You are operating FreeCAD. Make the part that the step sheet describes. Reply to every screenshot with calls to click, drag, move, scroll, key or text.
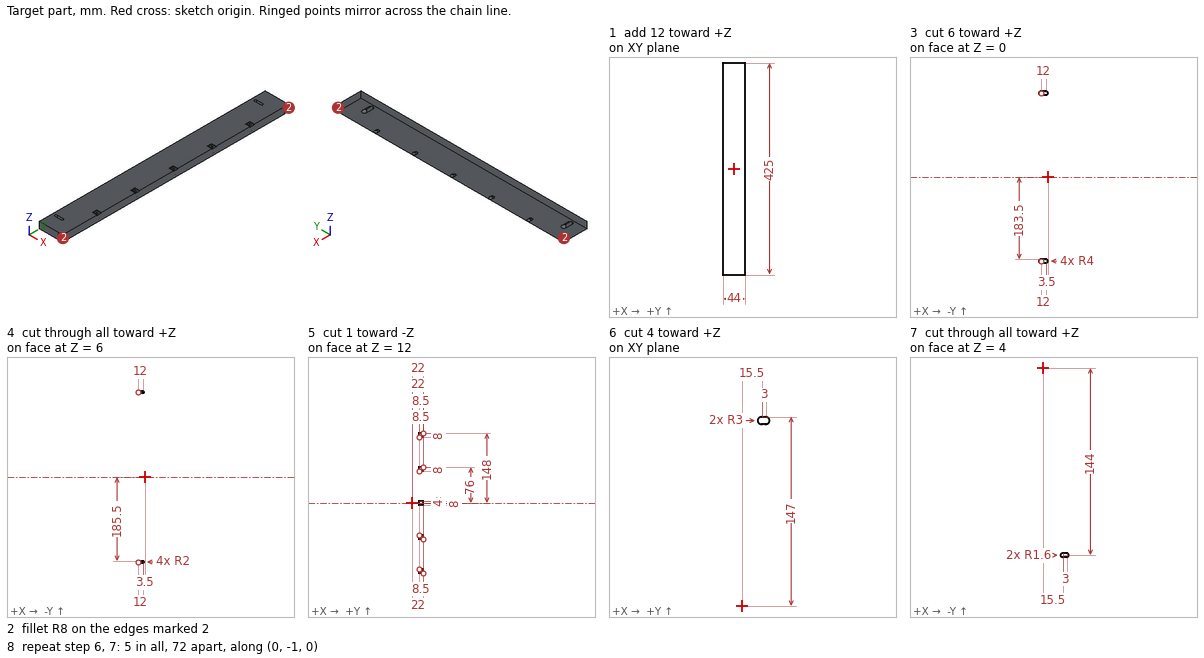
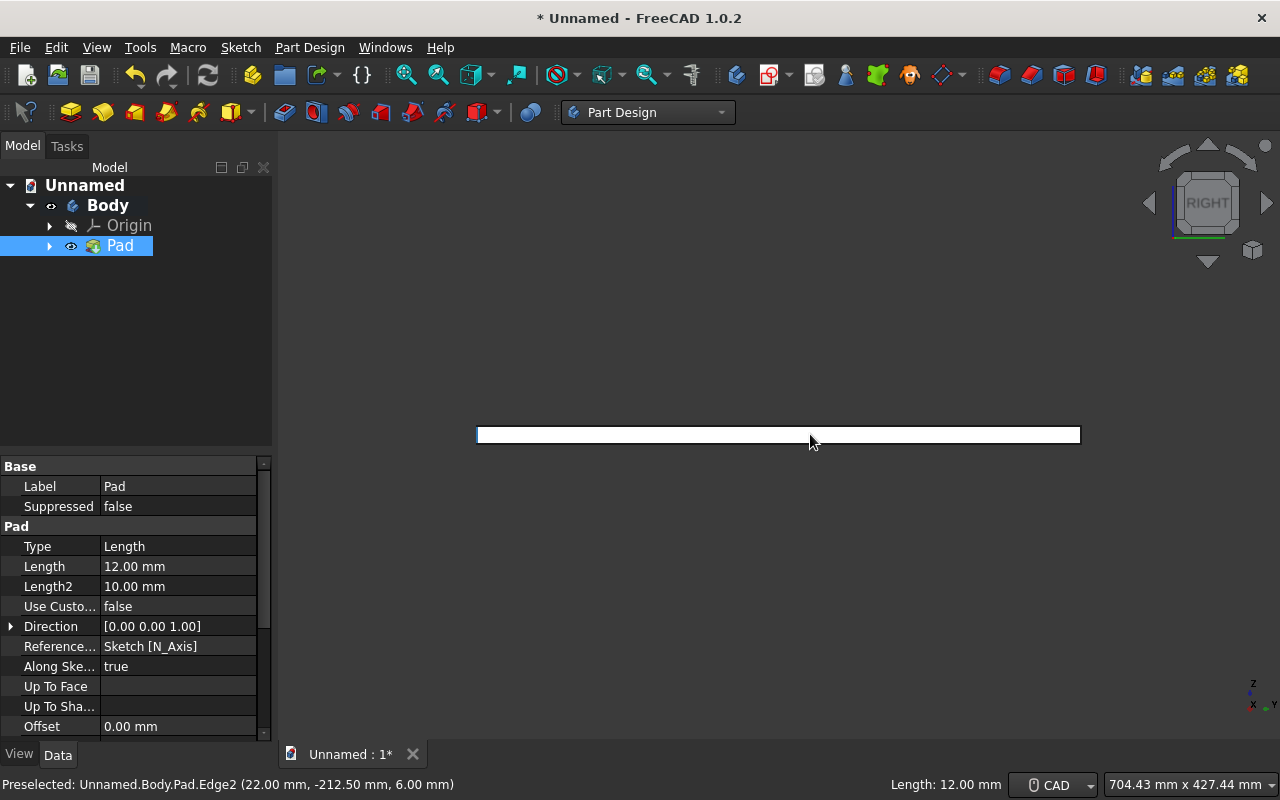
click(1081, 434, ctrl)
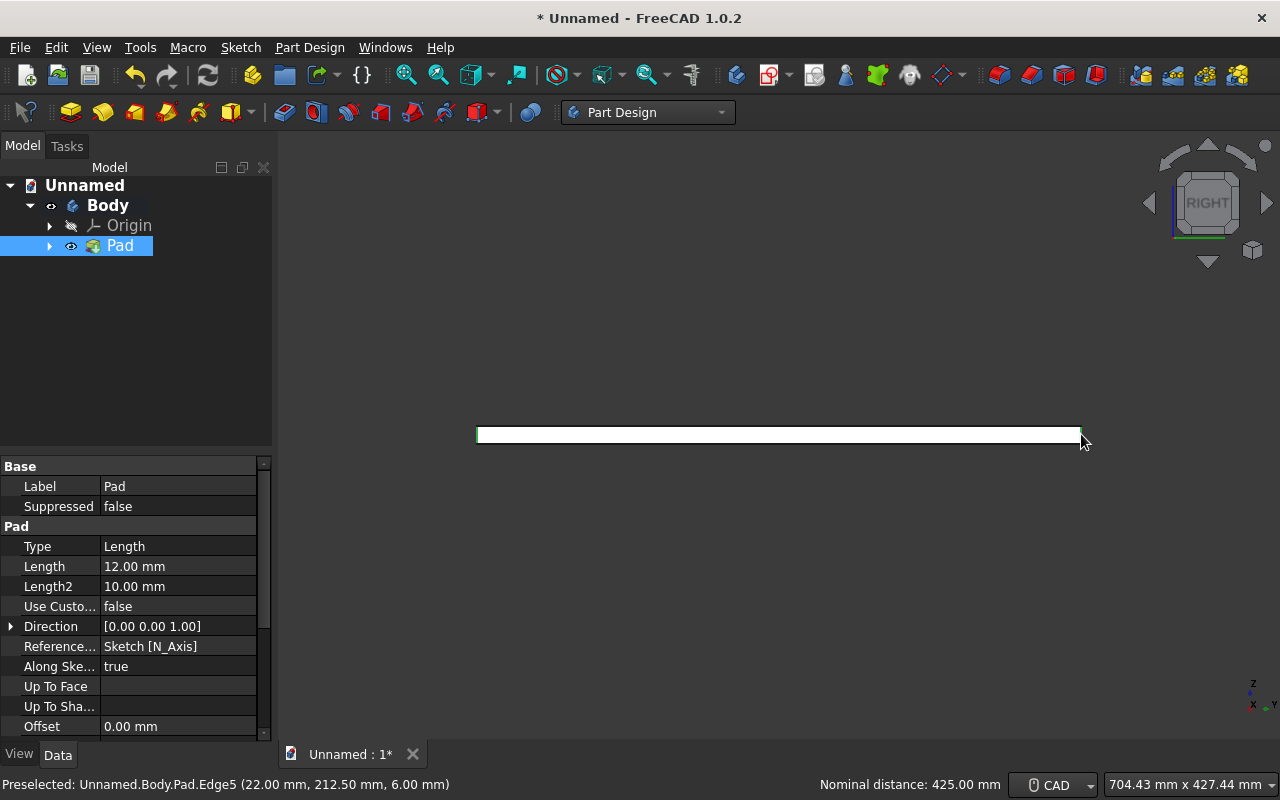
click(1000, 76)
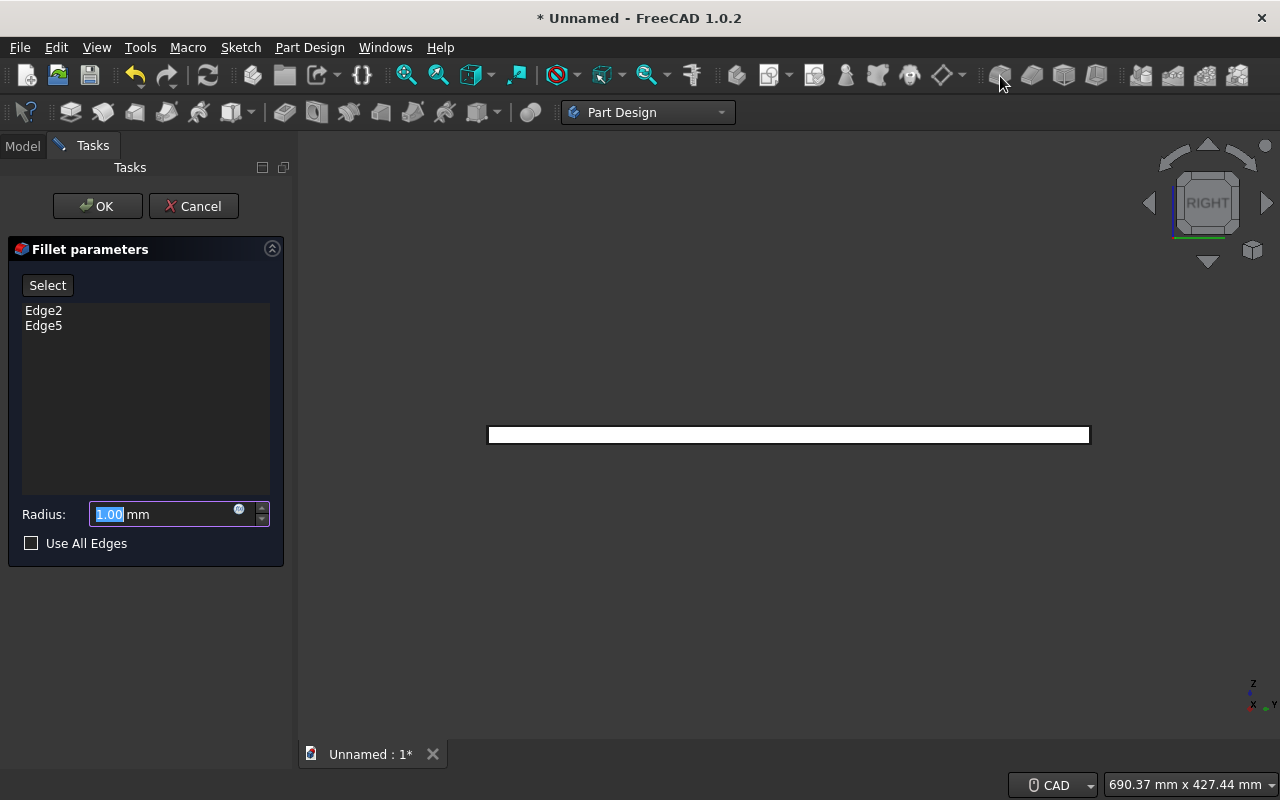
text(8)
key(Tab)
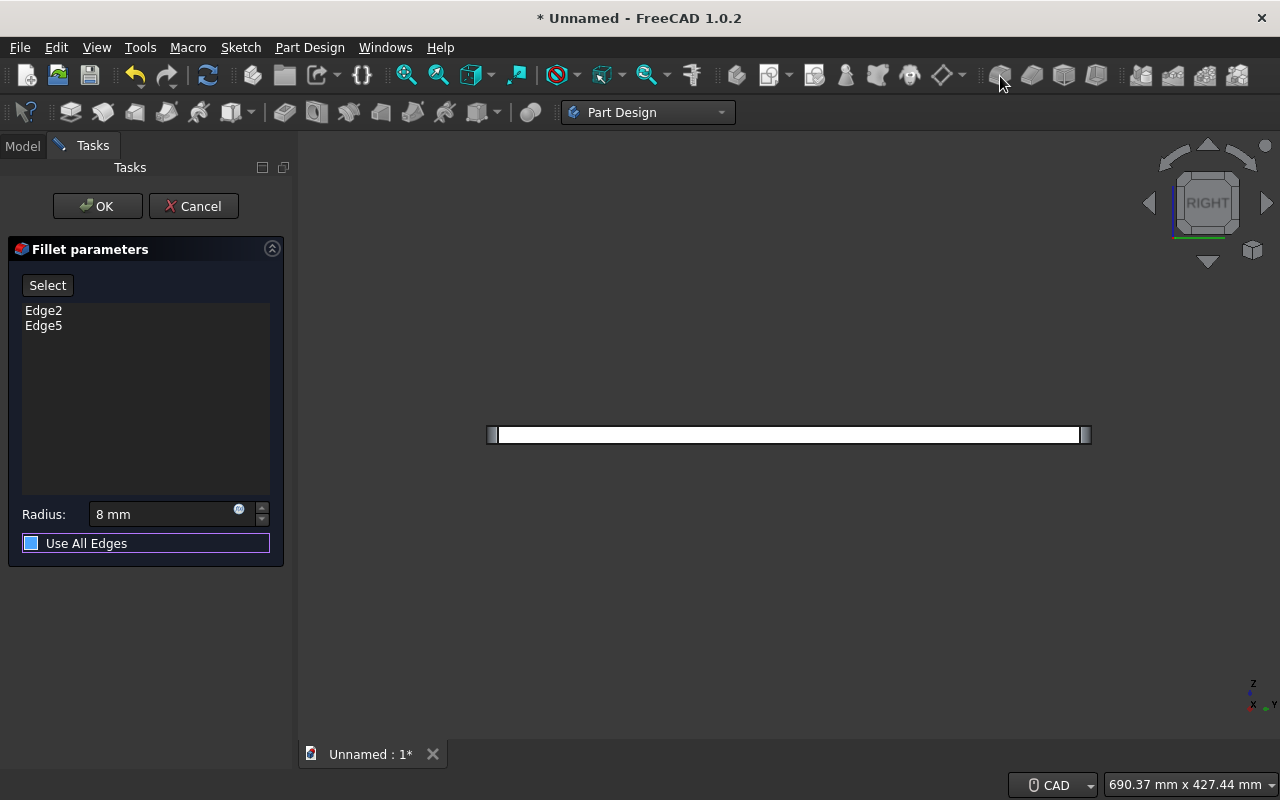
click(98, 206)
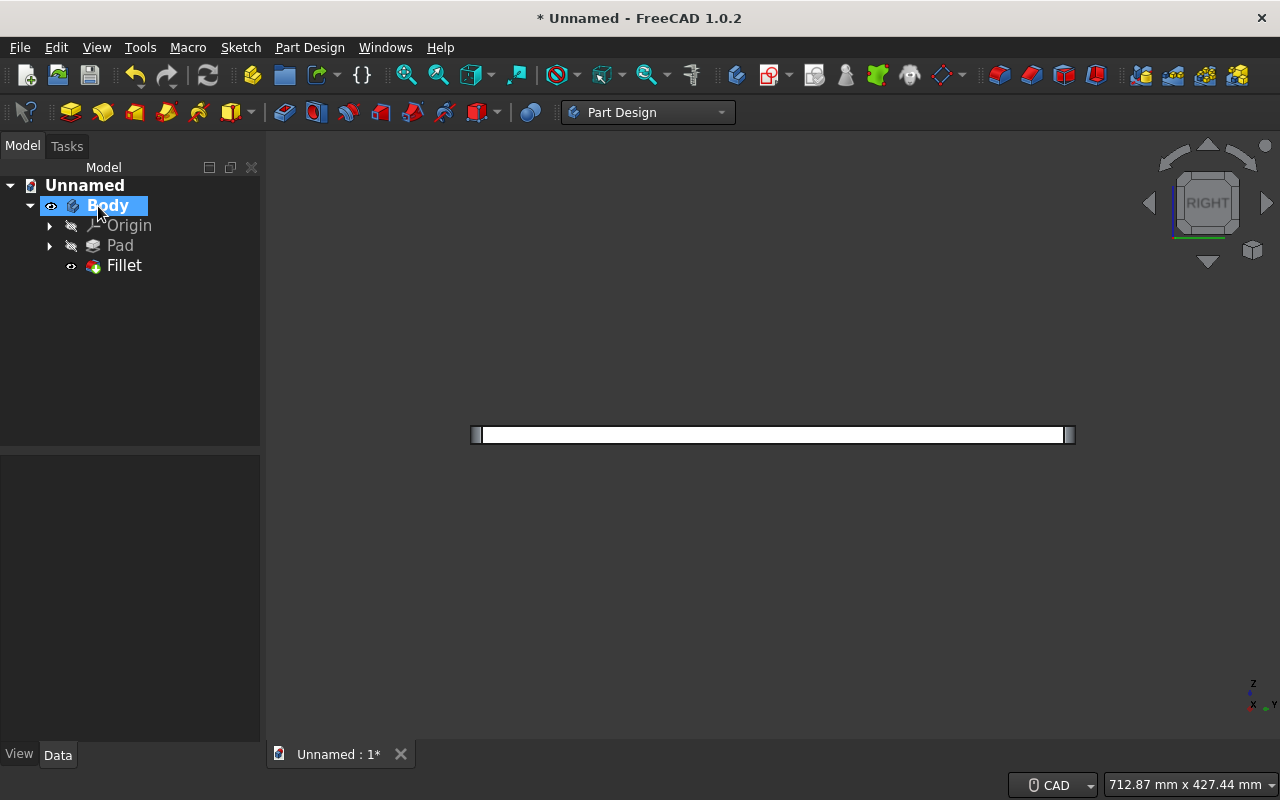
key(5)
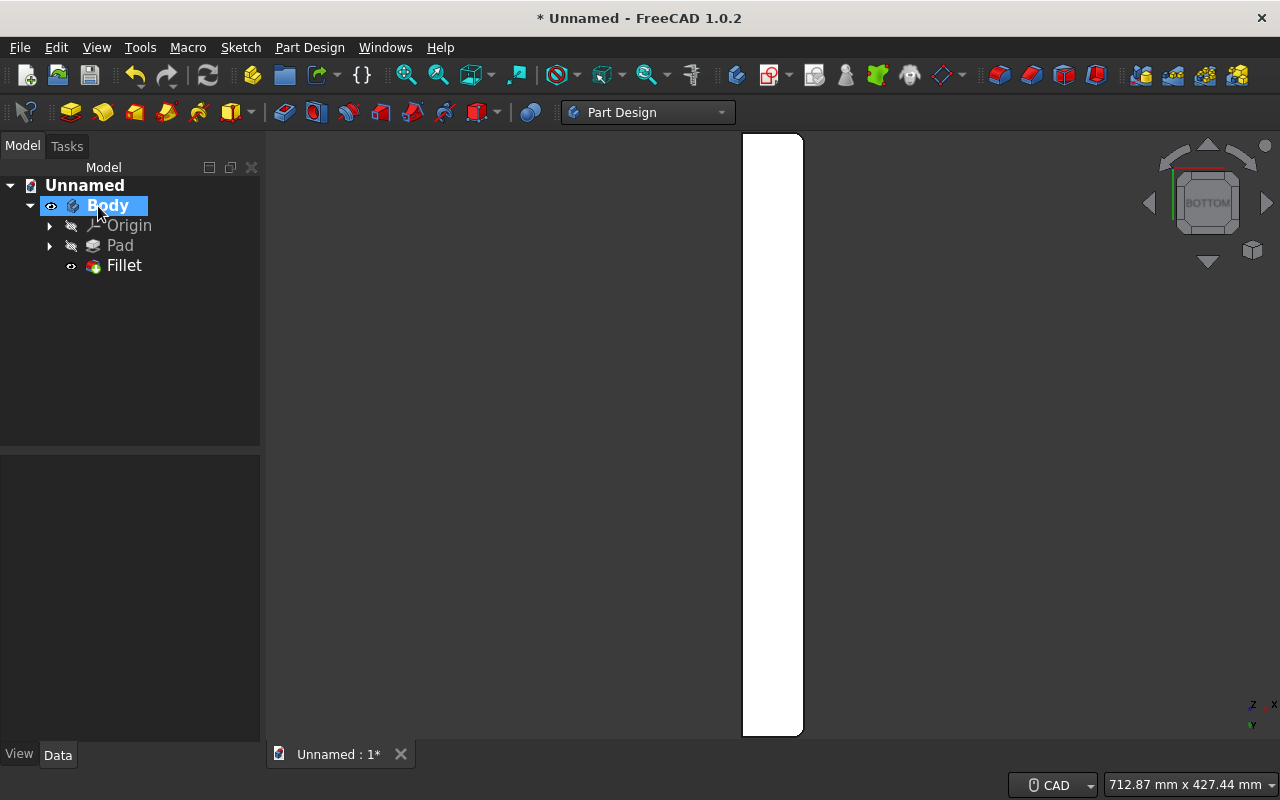
click(773, 693)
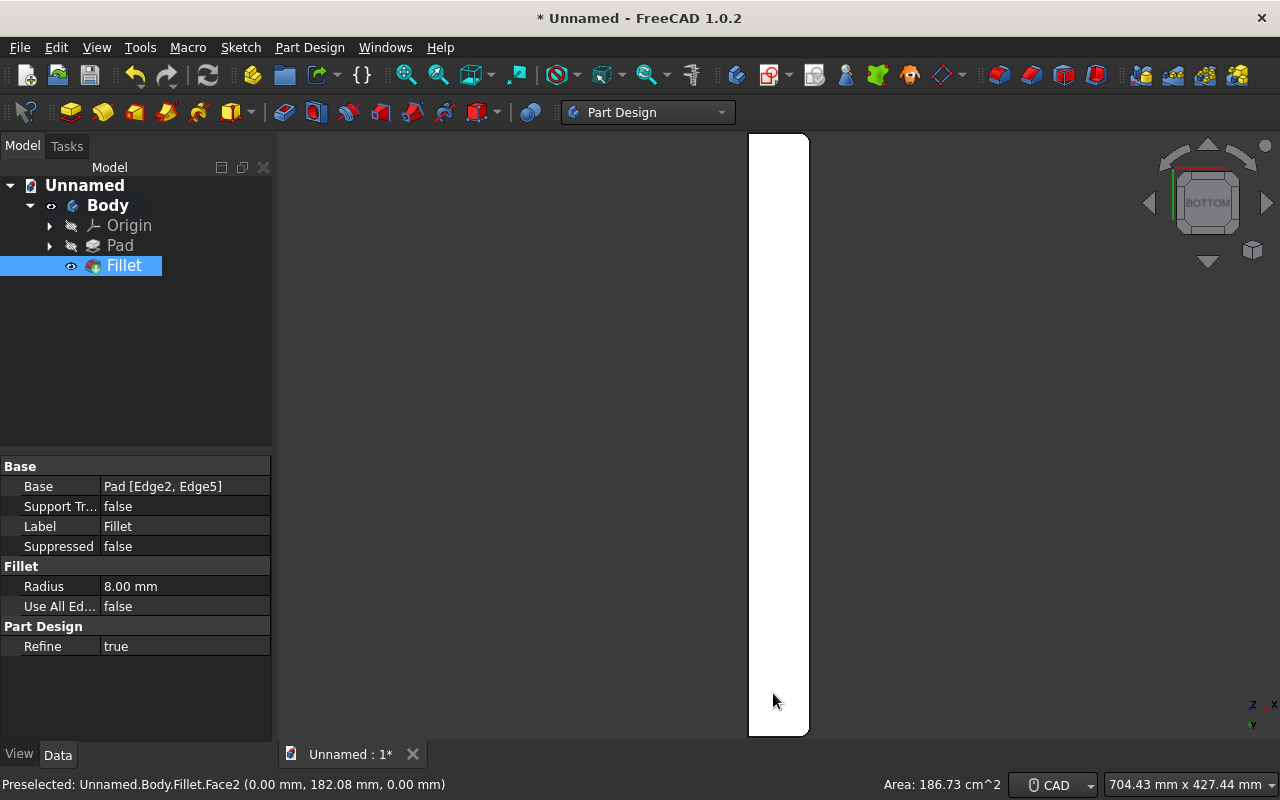
click(770, 76)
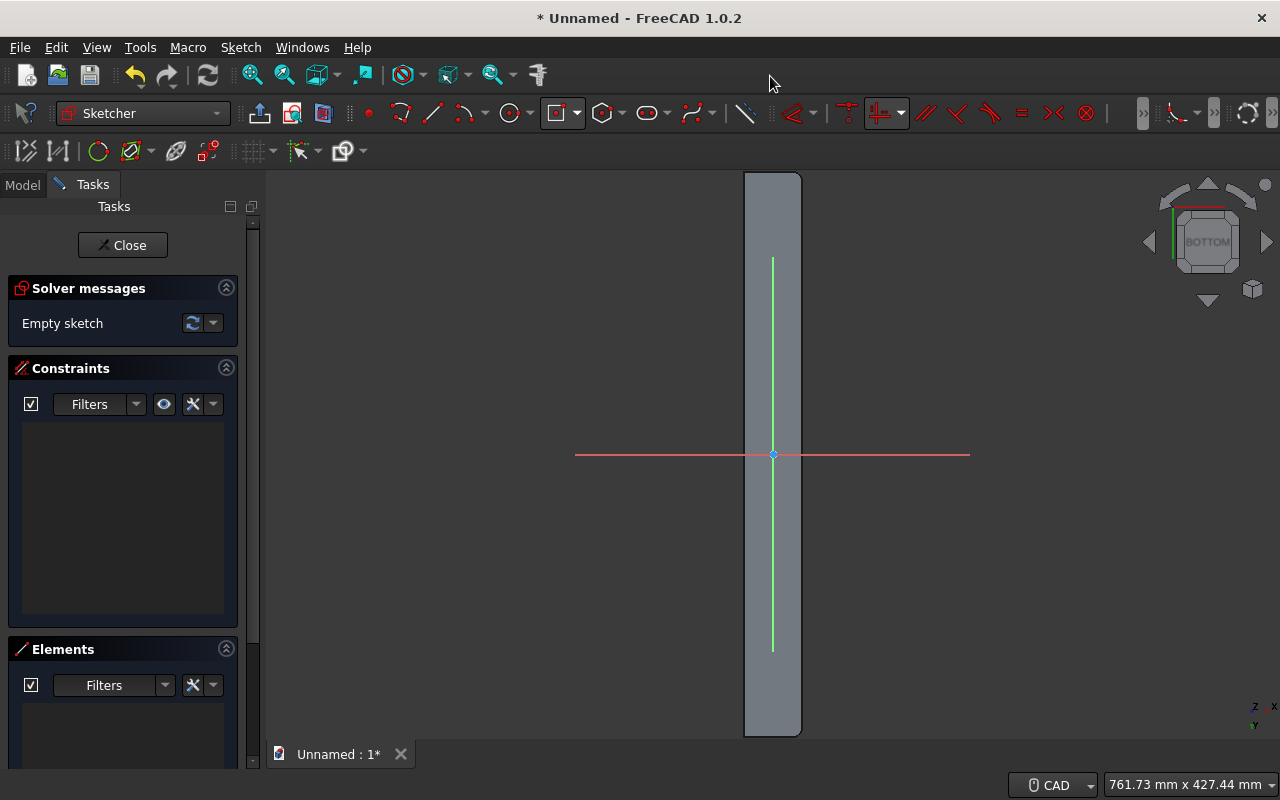
scroll(591, 455, down, 2)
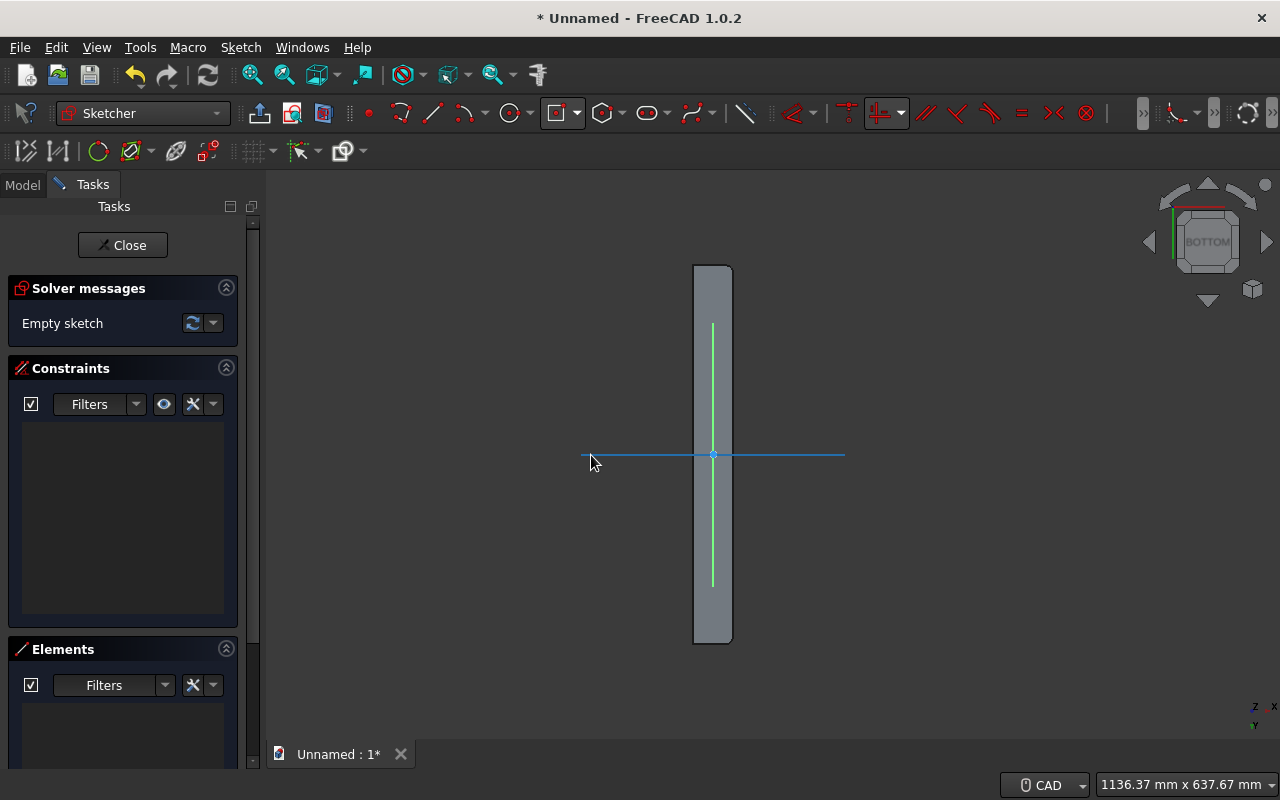
click(648, 114)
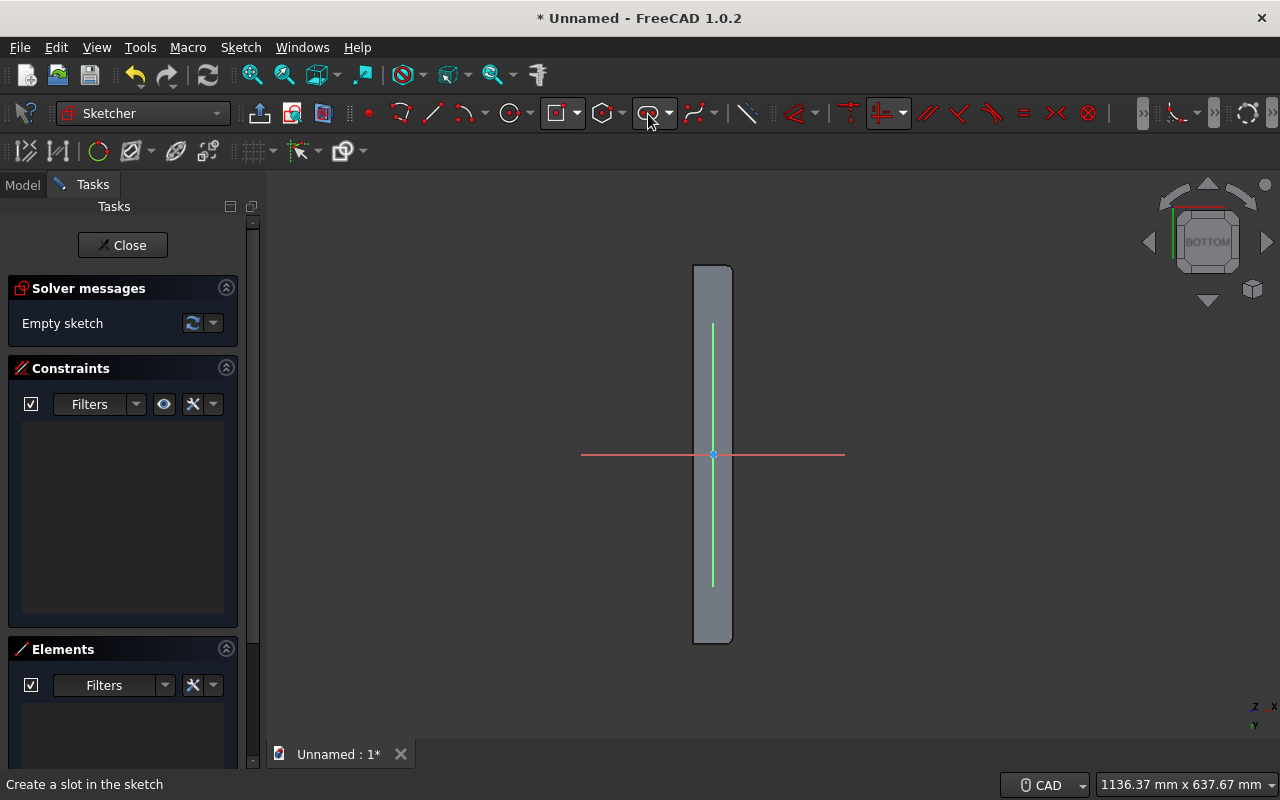
scroll(699, 622, up, 10)